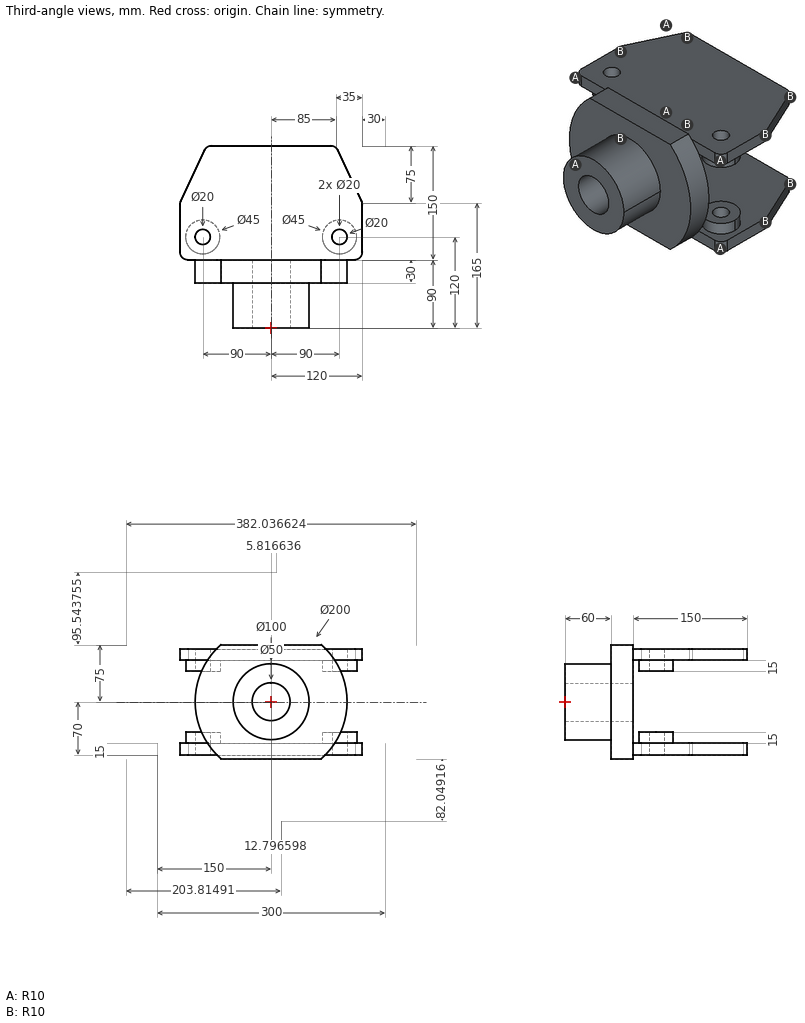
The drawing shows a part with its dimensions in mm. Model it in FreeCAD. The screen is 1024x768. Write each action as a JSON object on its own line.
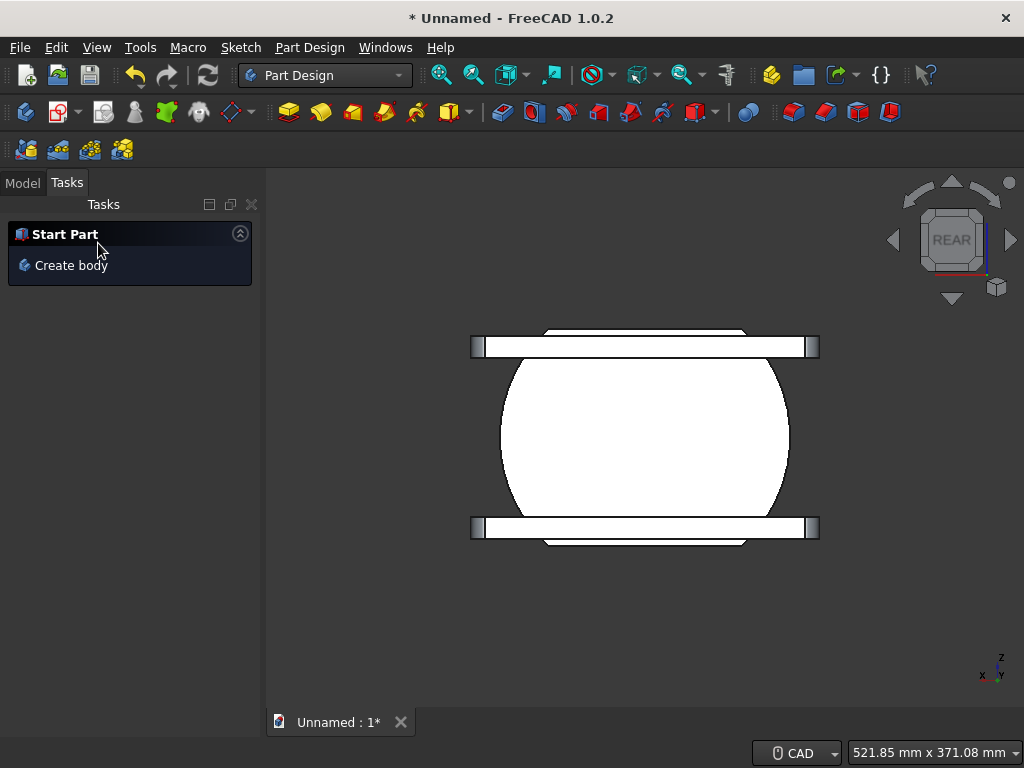
{"action": "left_click", "coordinate": [603, 437]}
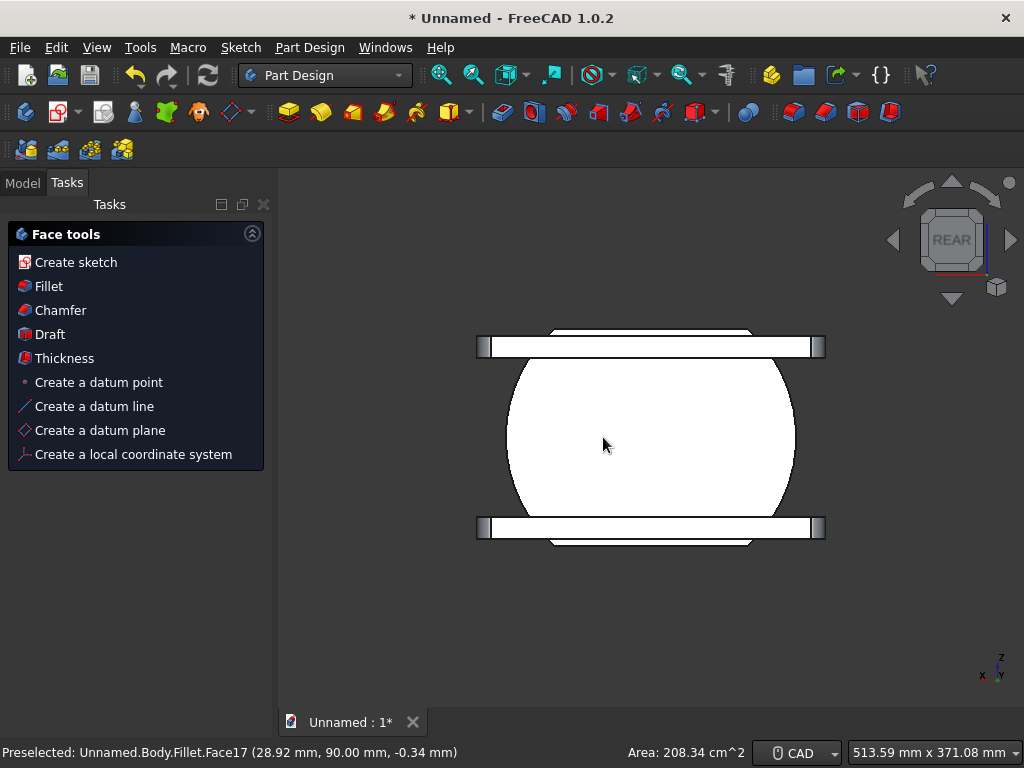
{"action": "left_click", "coordinate": [58, 112]}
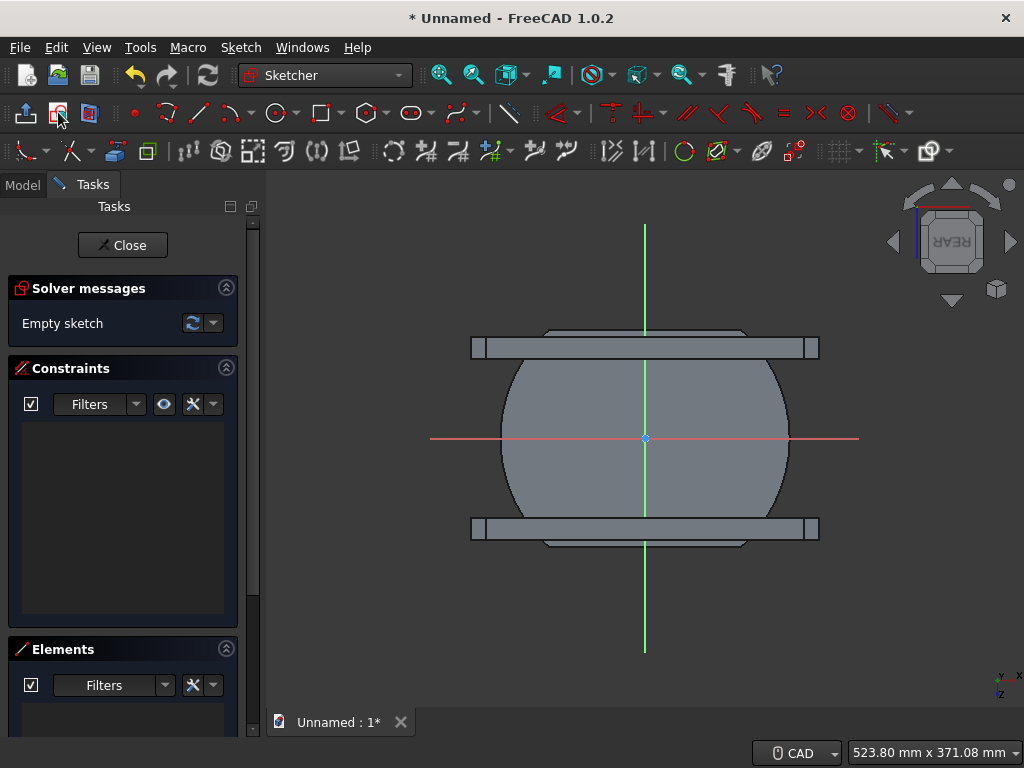
{"action": "left_click", "coordinate": [90, 114]}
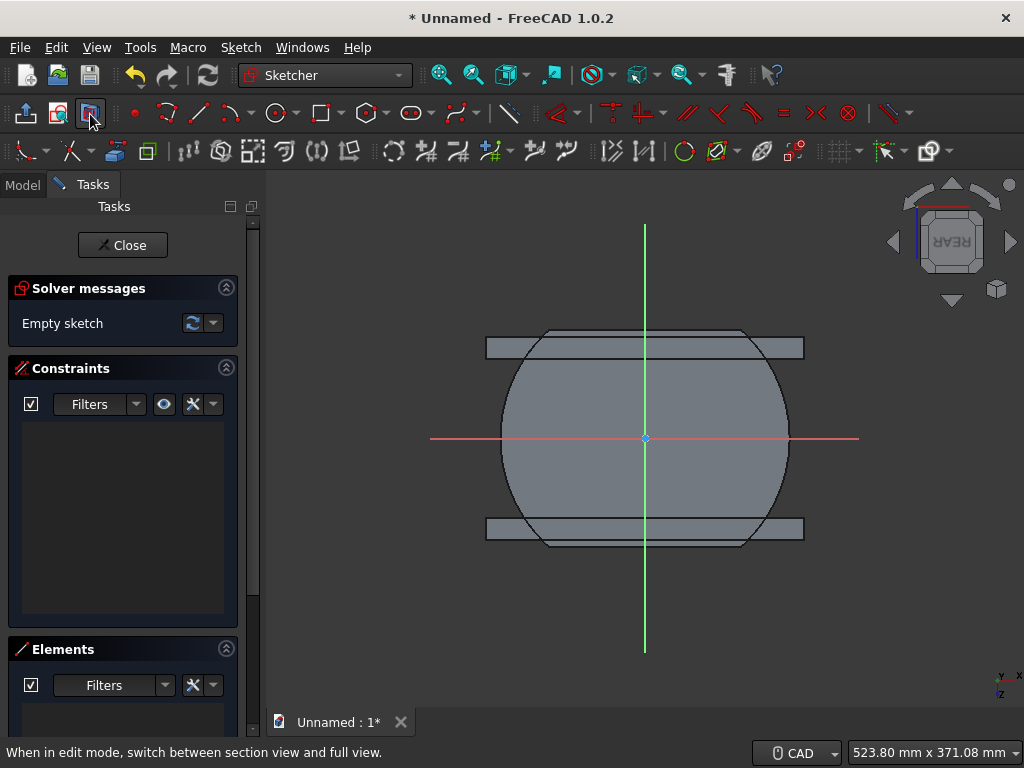
{"action": "scroll", "coordinate": [662, 438], "scroll_direction": "up", "scroll_amount": 8}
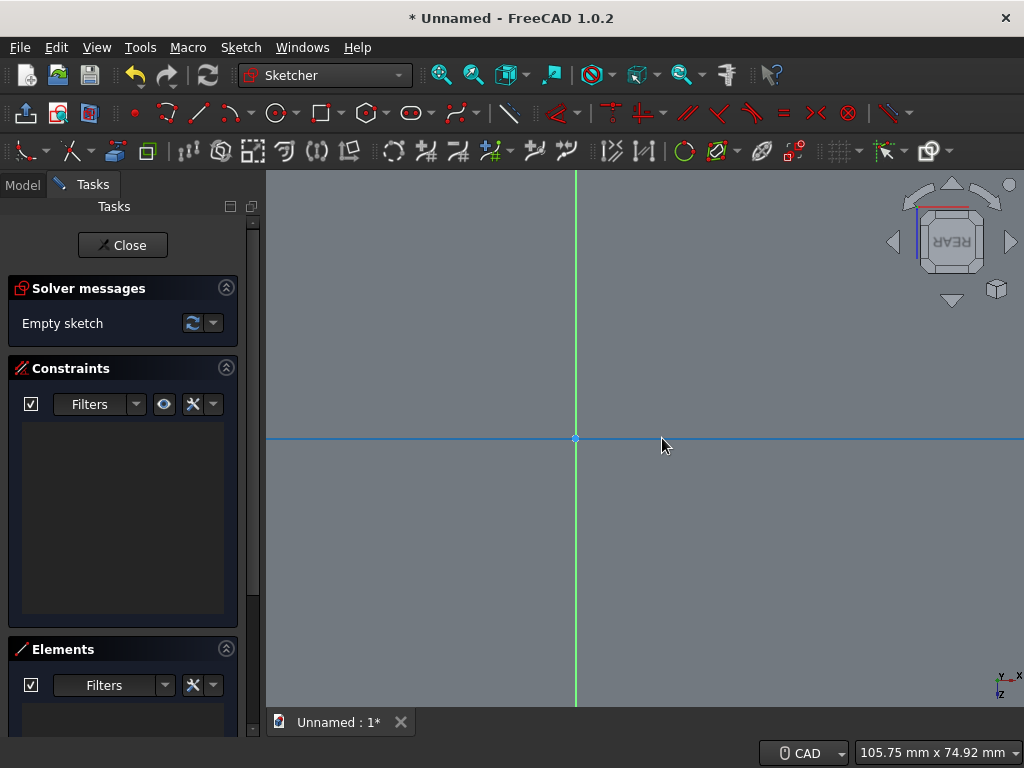
{"action": "left_click", "coordinate": [276, 114]}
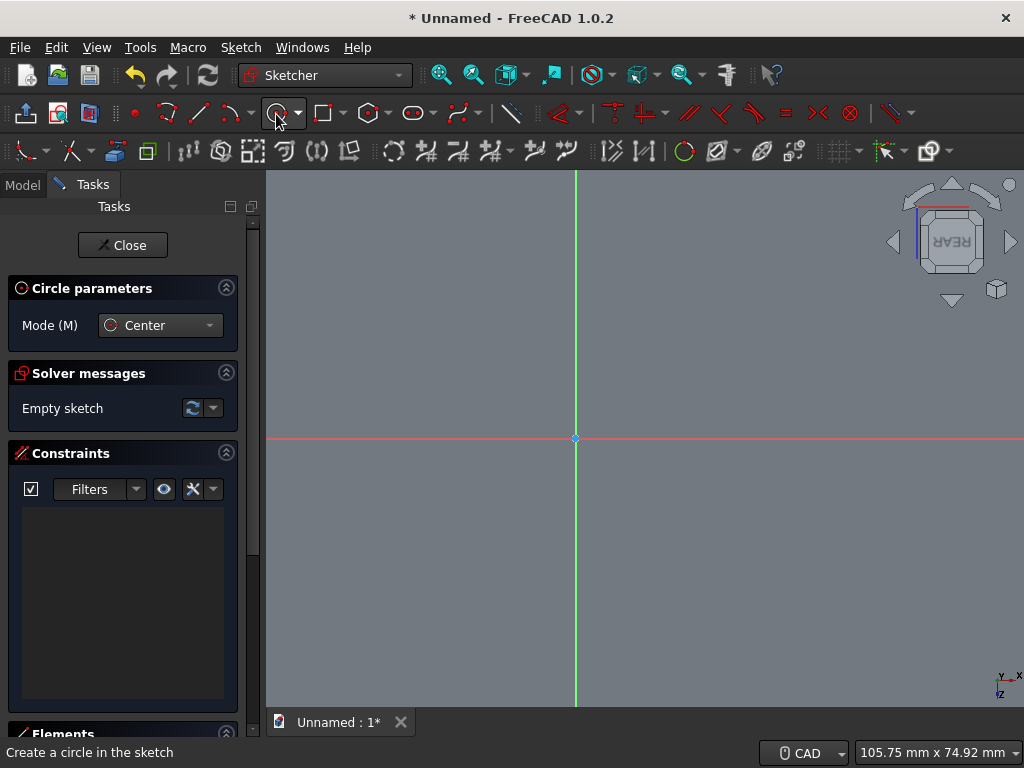
{"action": "left_click", "coordinate": [576, 438]}
{"action": "left_click", "coordinate": [702, 312]}
{"action": "key", "text": "Escape"}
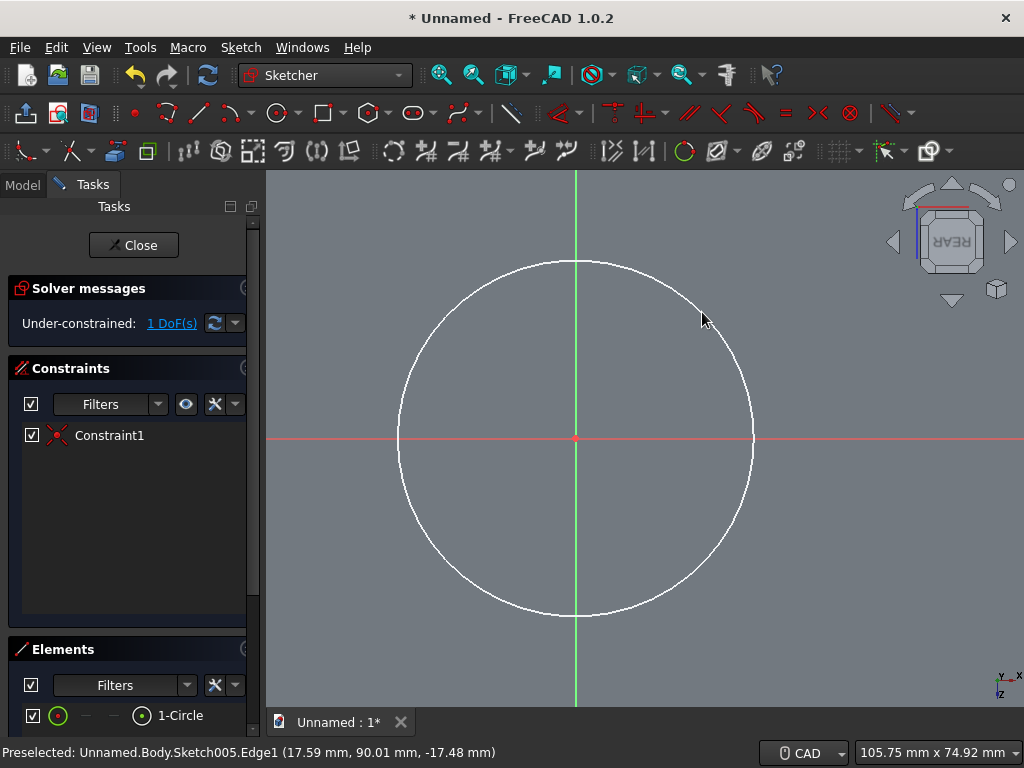
{"action": "left_click", "coordinate": [558, 114]}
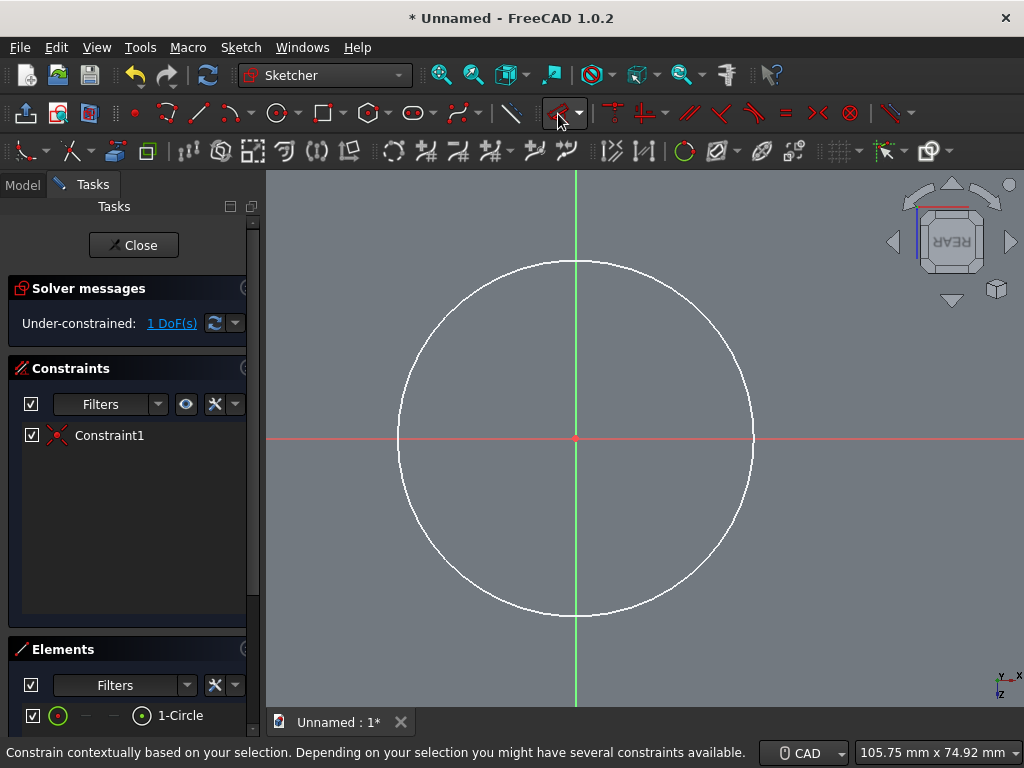
{"action": "left_click", "coordinate": [701, 312]}
{"action": "left_click", "coordinate": [724, 289]}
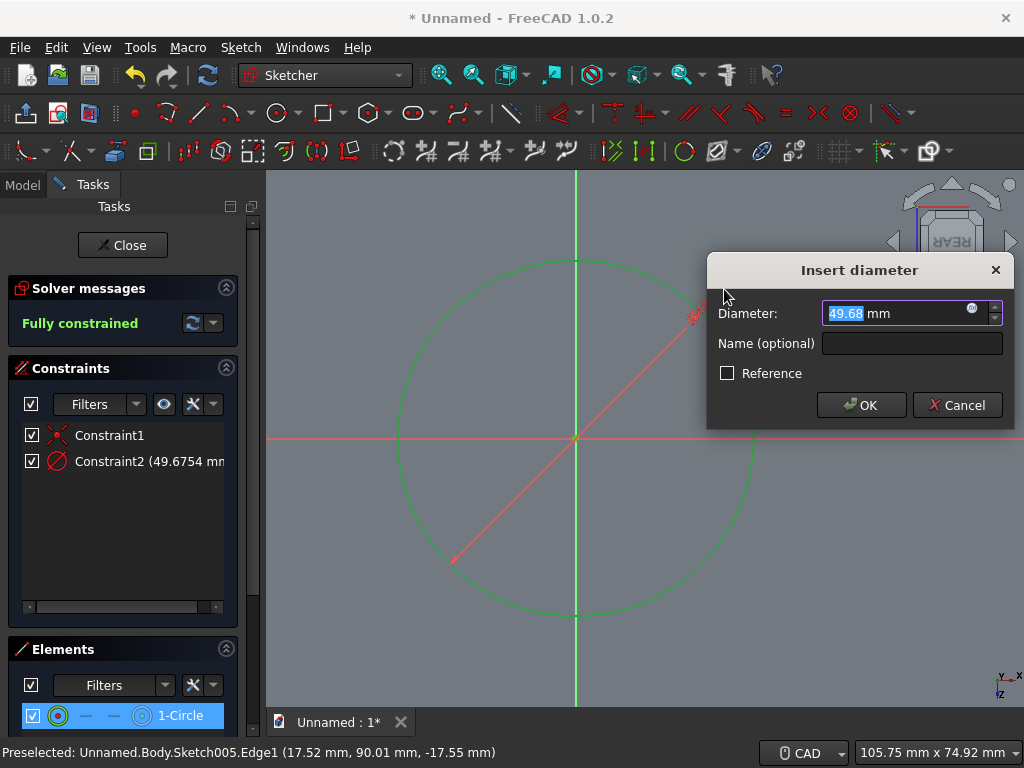
{"action": "type", "text": "50"}
{"action": "key", "text": "Return"}
{"action": "key", "text": "Escape"}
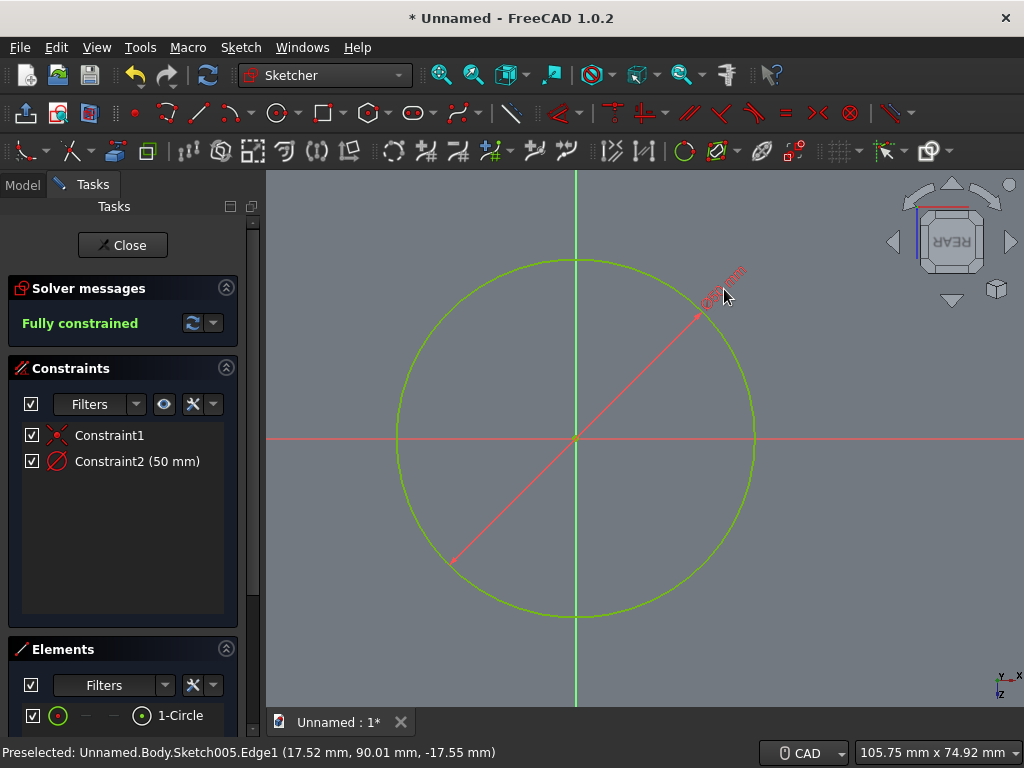
{"action": "left_click", "coordinate": [123, 245]}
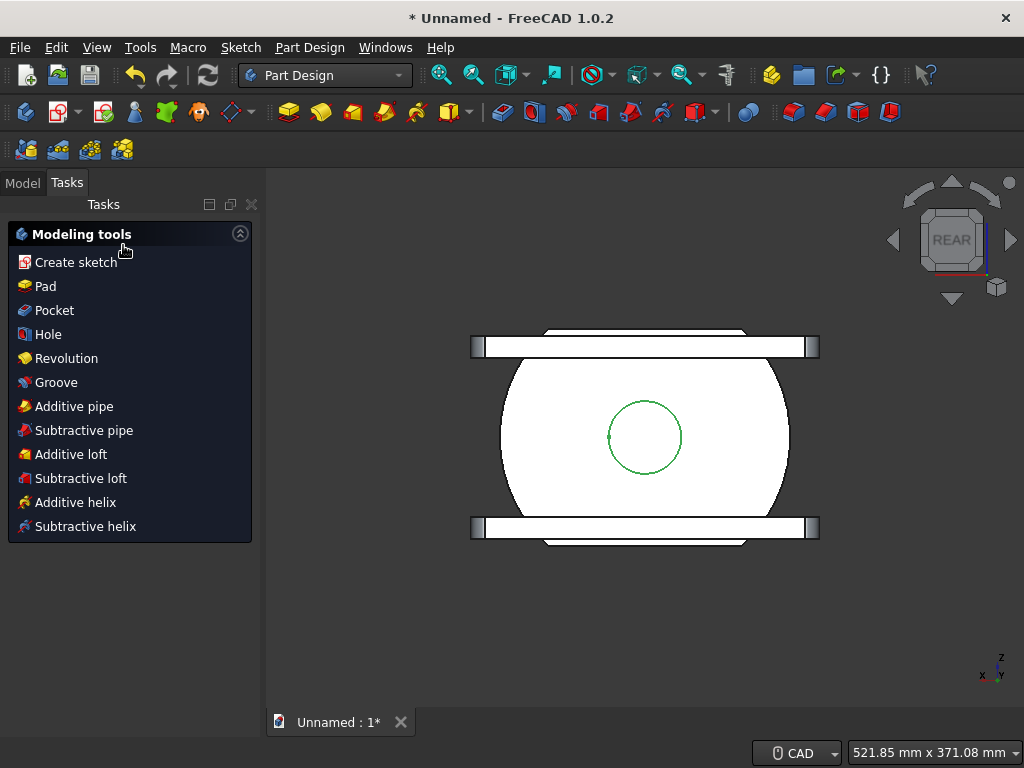
{"action": "left_click", "coordinate": [504, 112]}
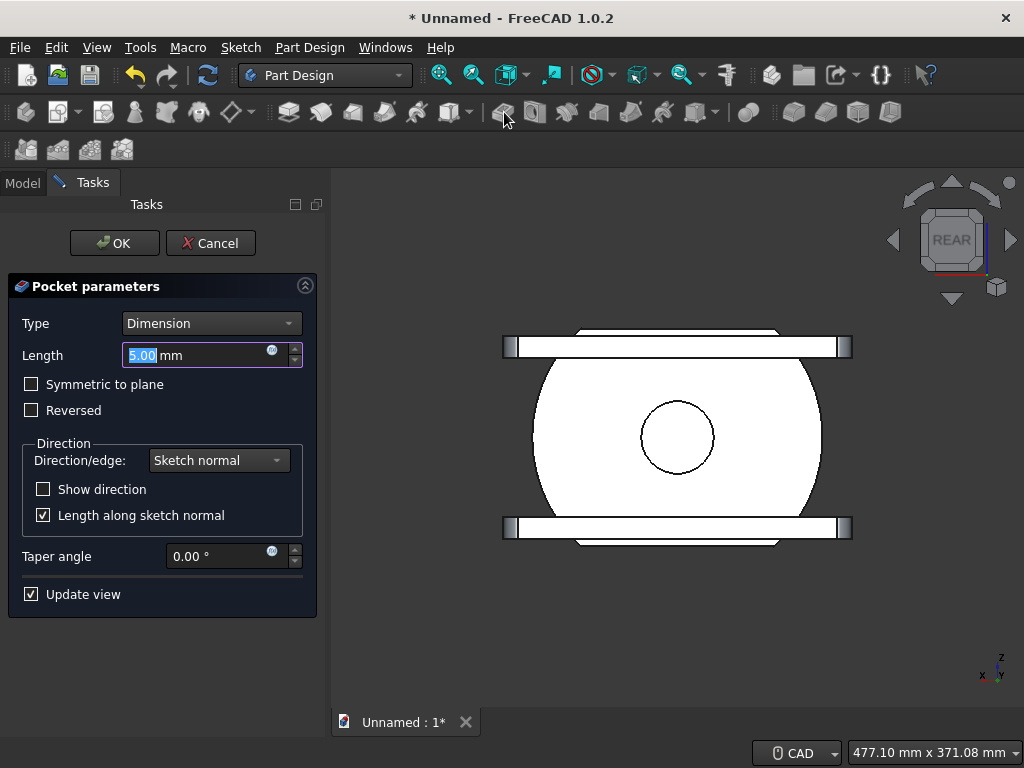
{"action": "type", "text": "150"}
{"action": "key", "text": "Tab"}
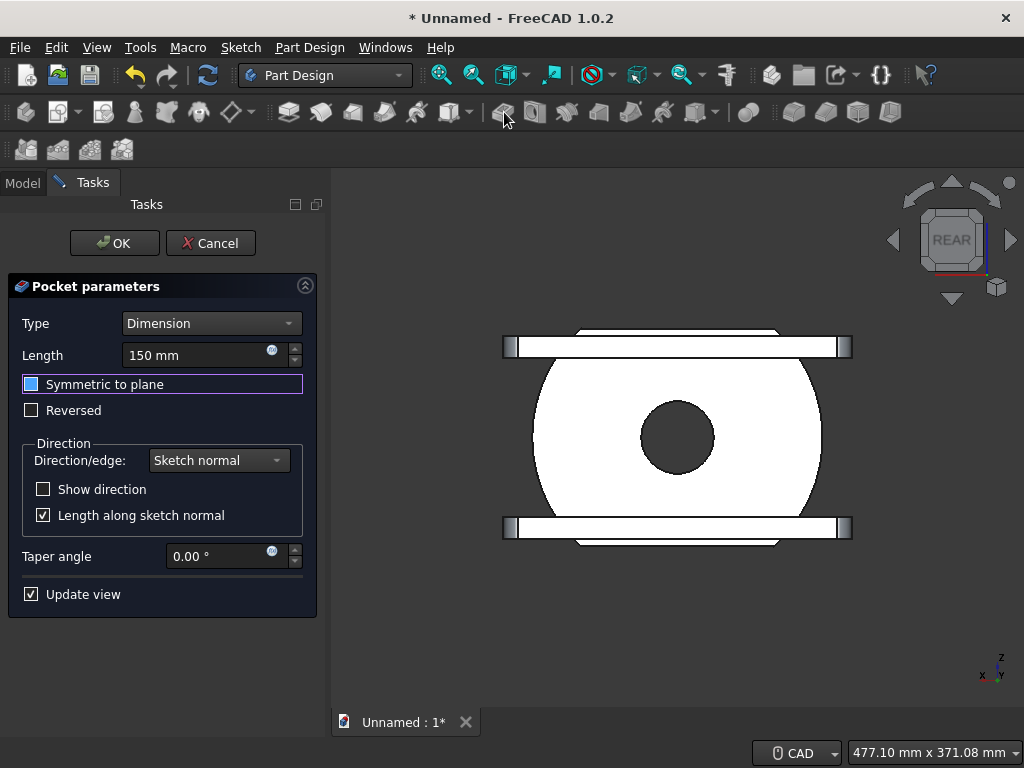
{"action": "left_click", "coordinate": [115, 243]}